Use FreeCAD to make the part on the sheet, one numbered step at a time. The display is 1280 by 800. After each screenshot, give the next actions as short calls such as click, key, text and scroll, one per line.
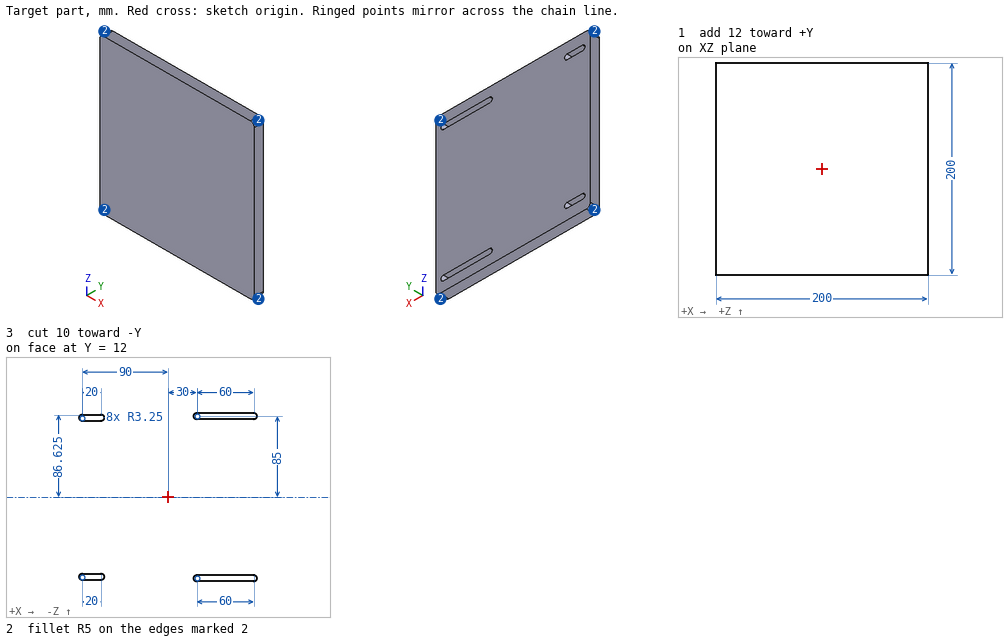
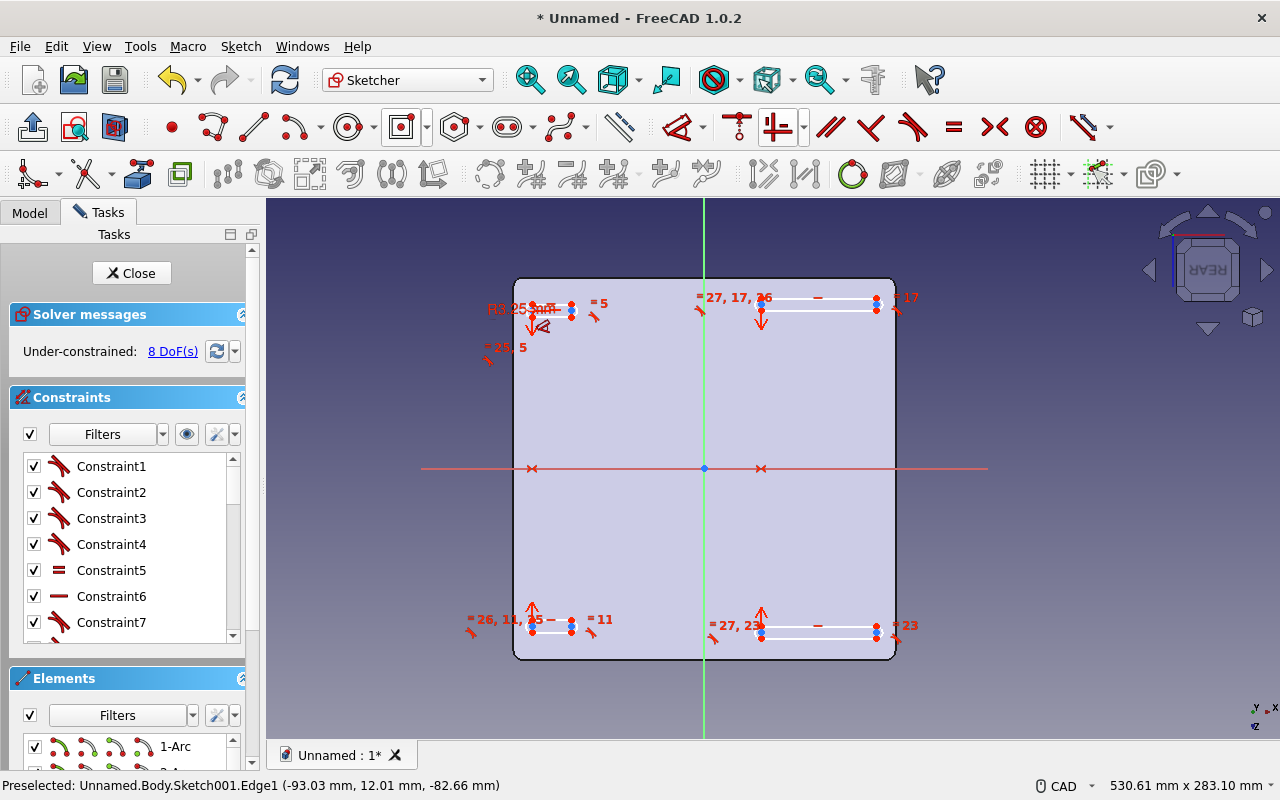
click(544, 305)
click(552, 271)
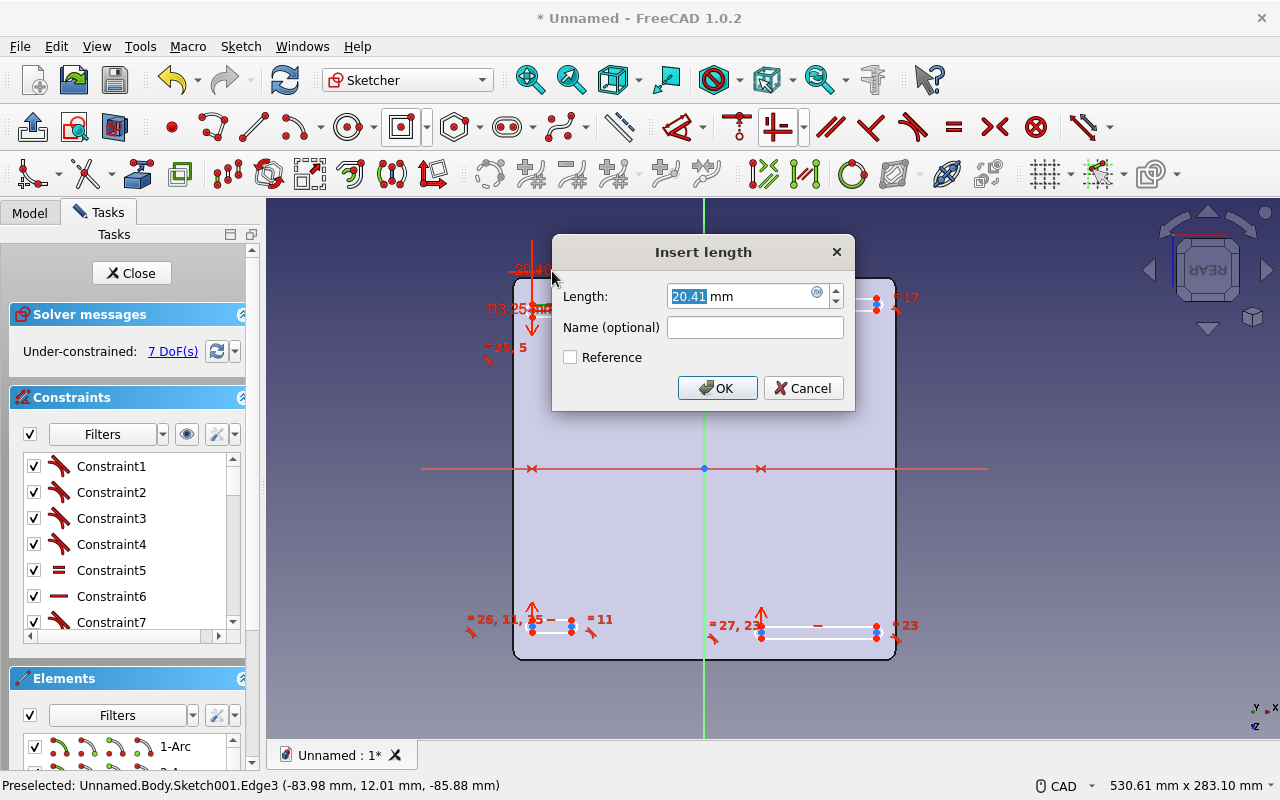
text(20)
key(Return)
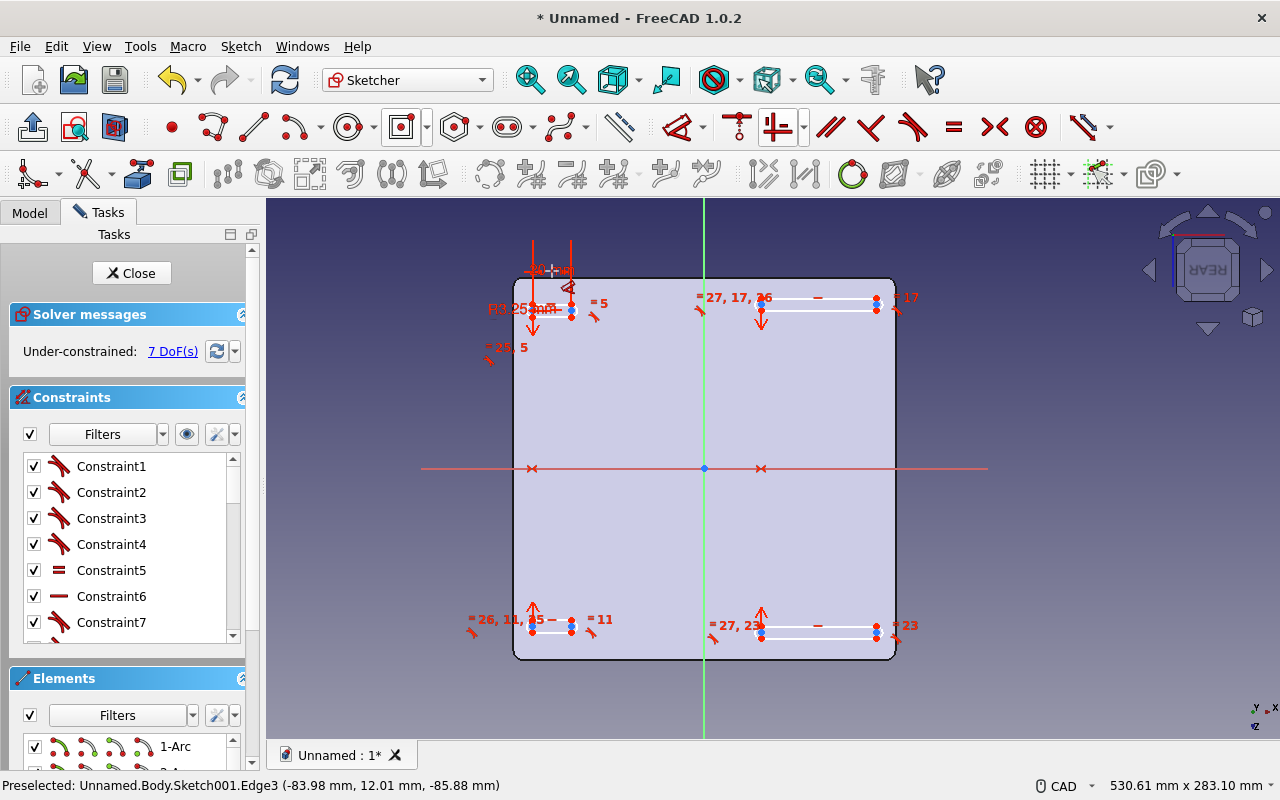
click(544, 620)
click(552, 654)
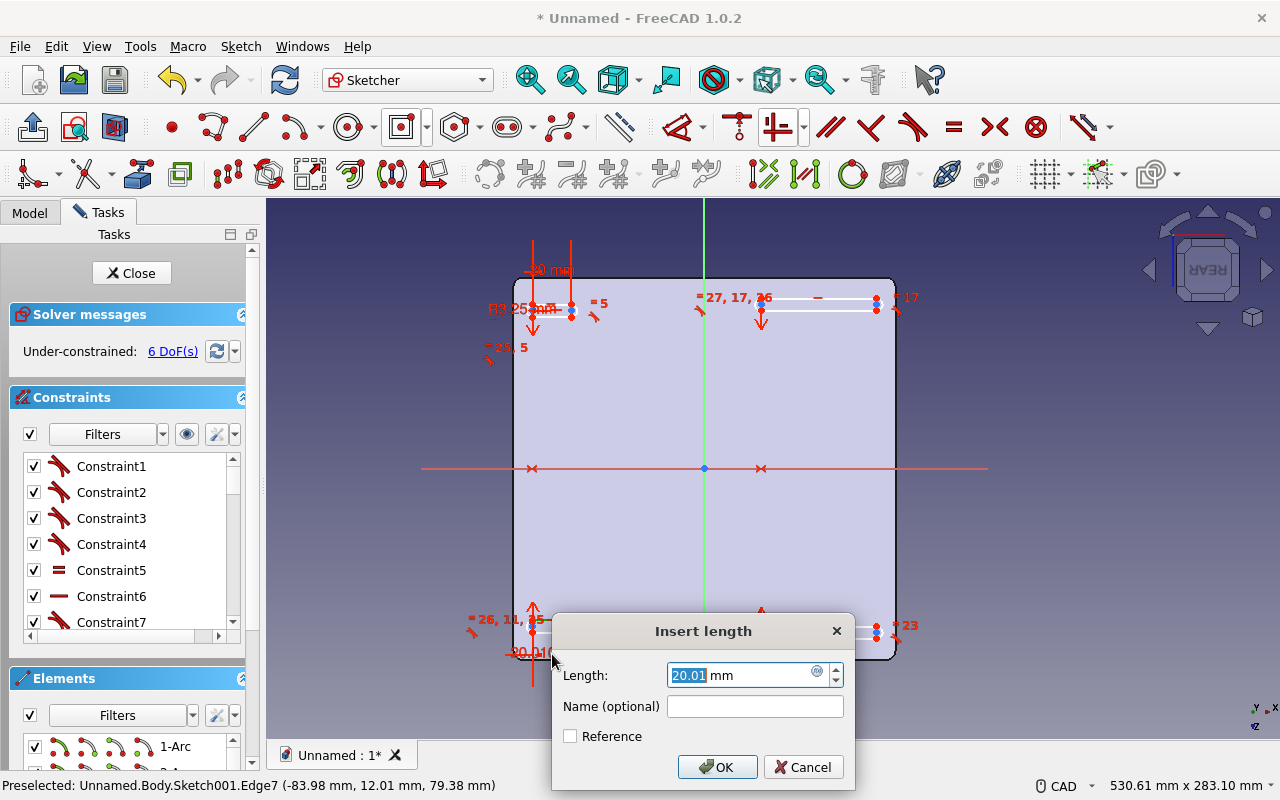
text(20)
key(Return)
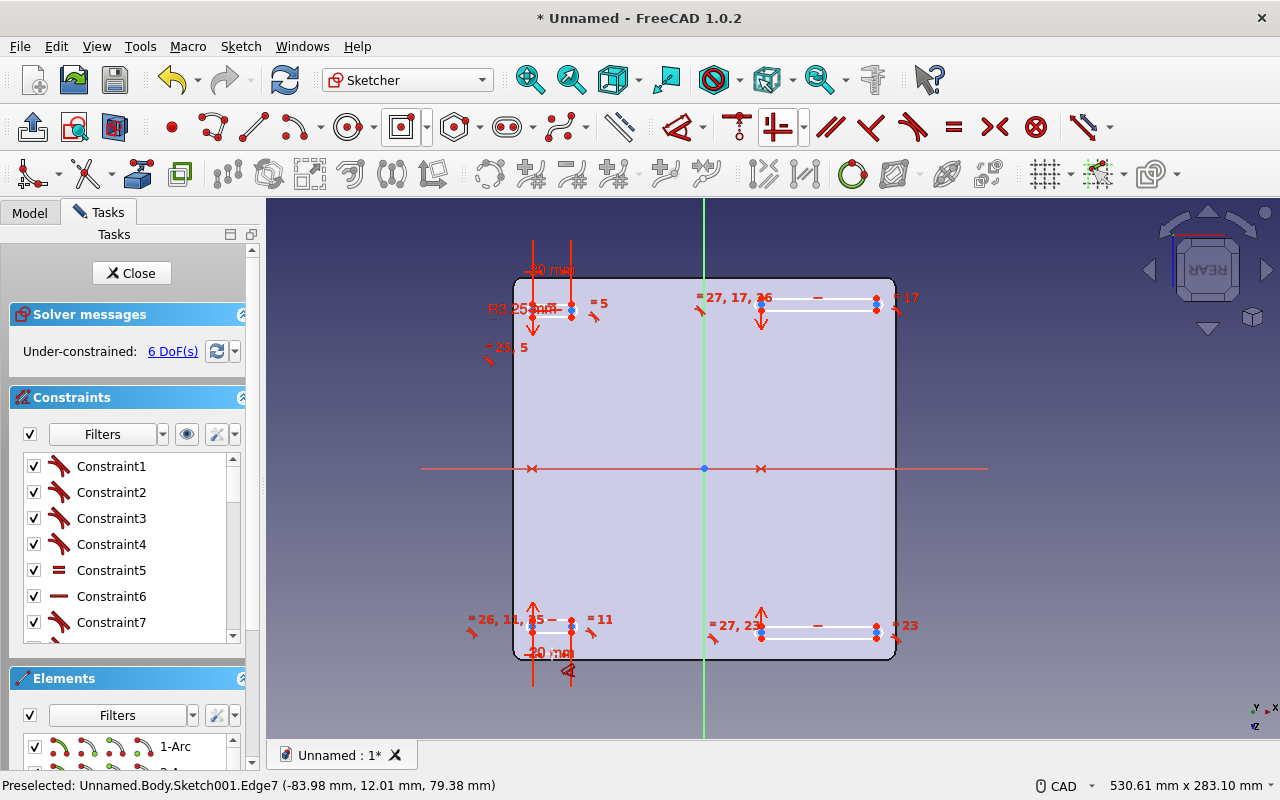
click(796, 299)
click(819, 265)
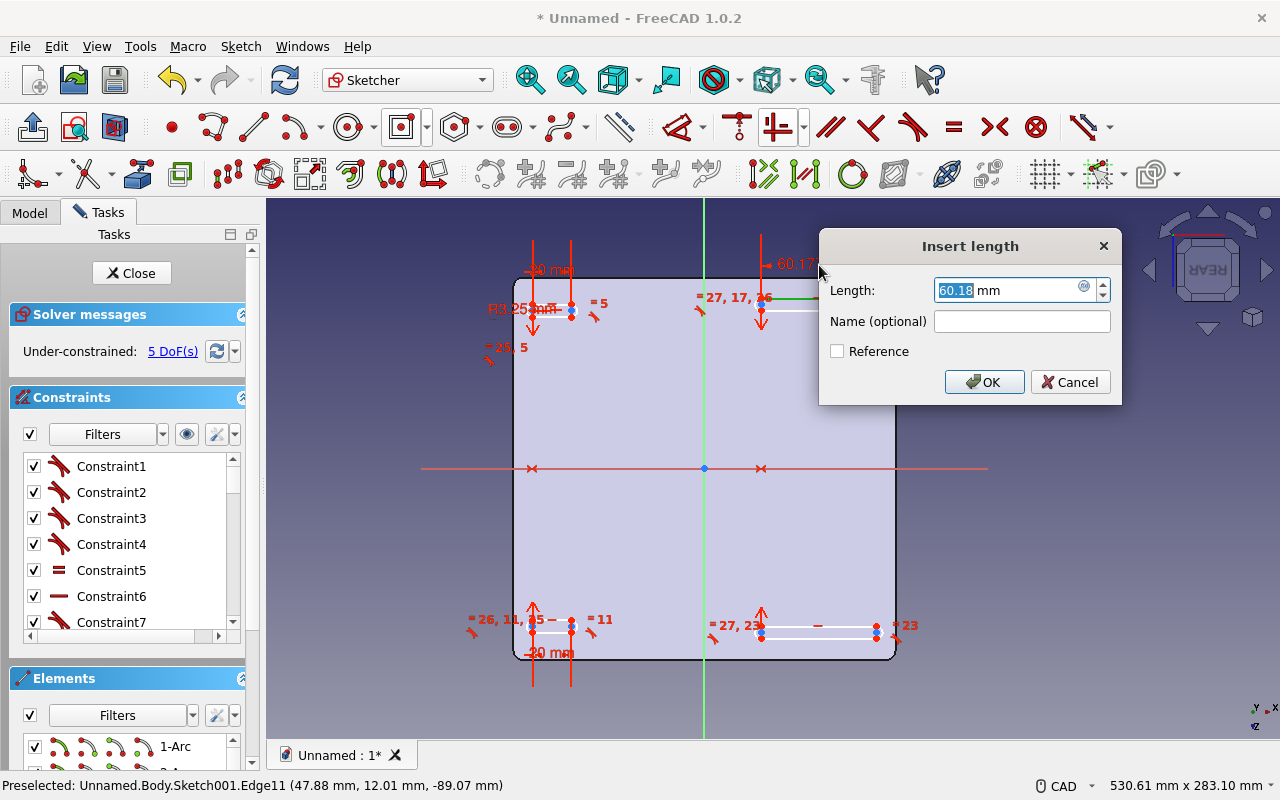
text(60)
key(Return)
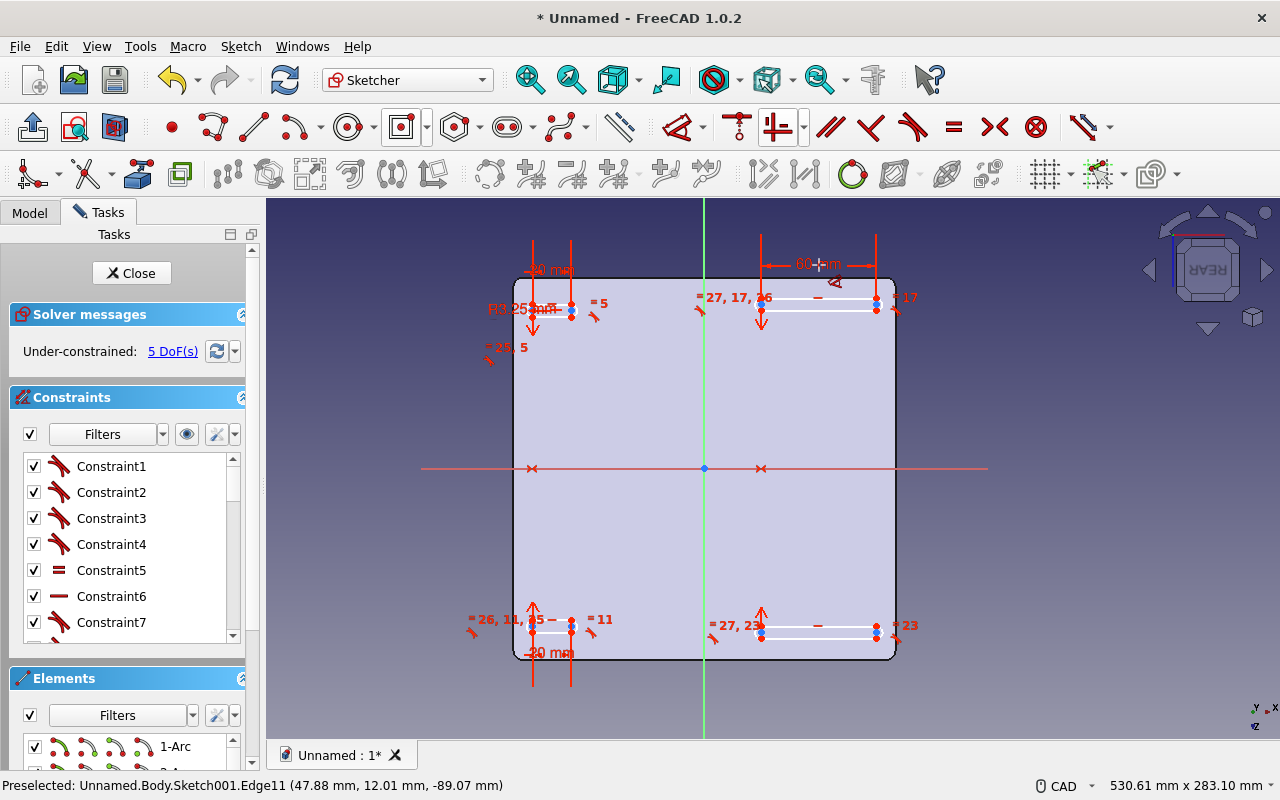
click(796, 627)
click(819, 661)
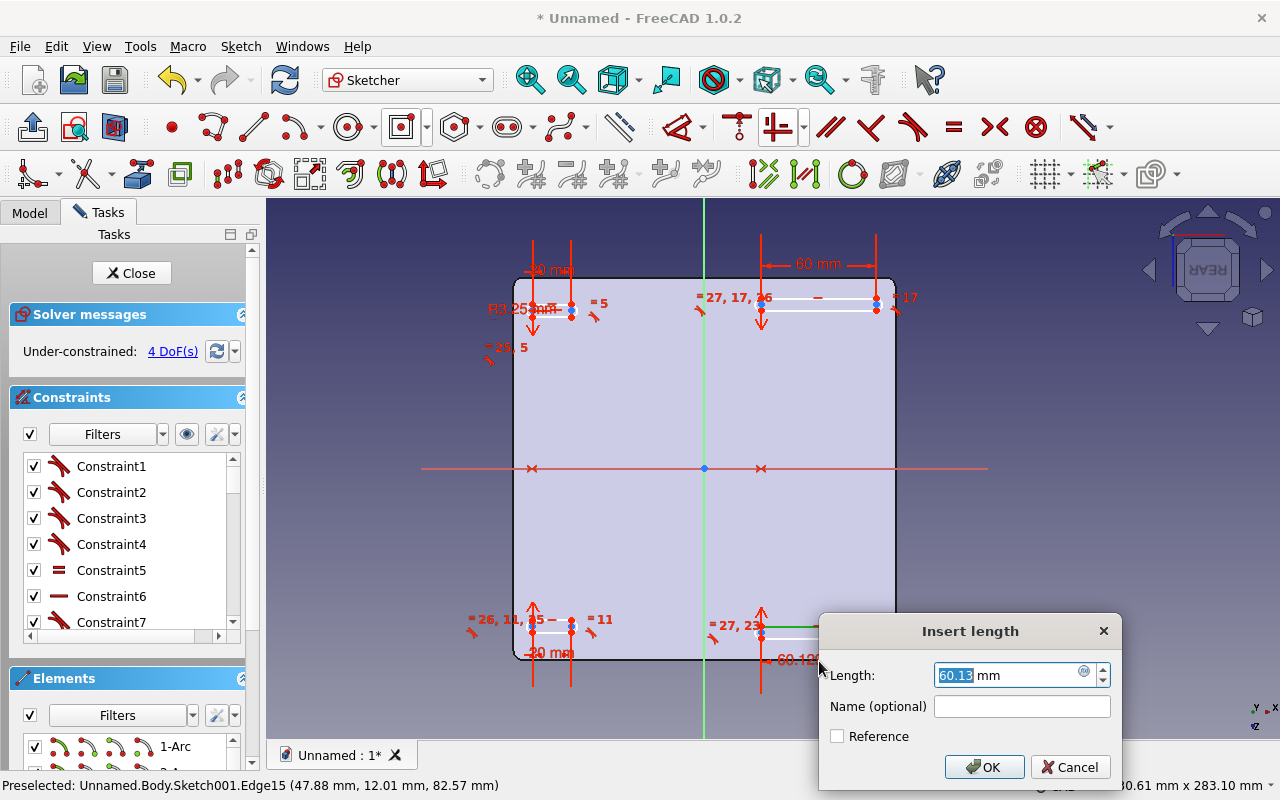
text(60)
key(Return)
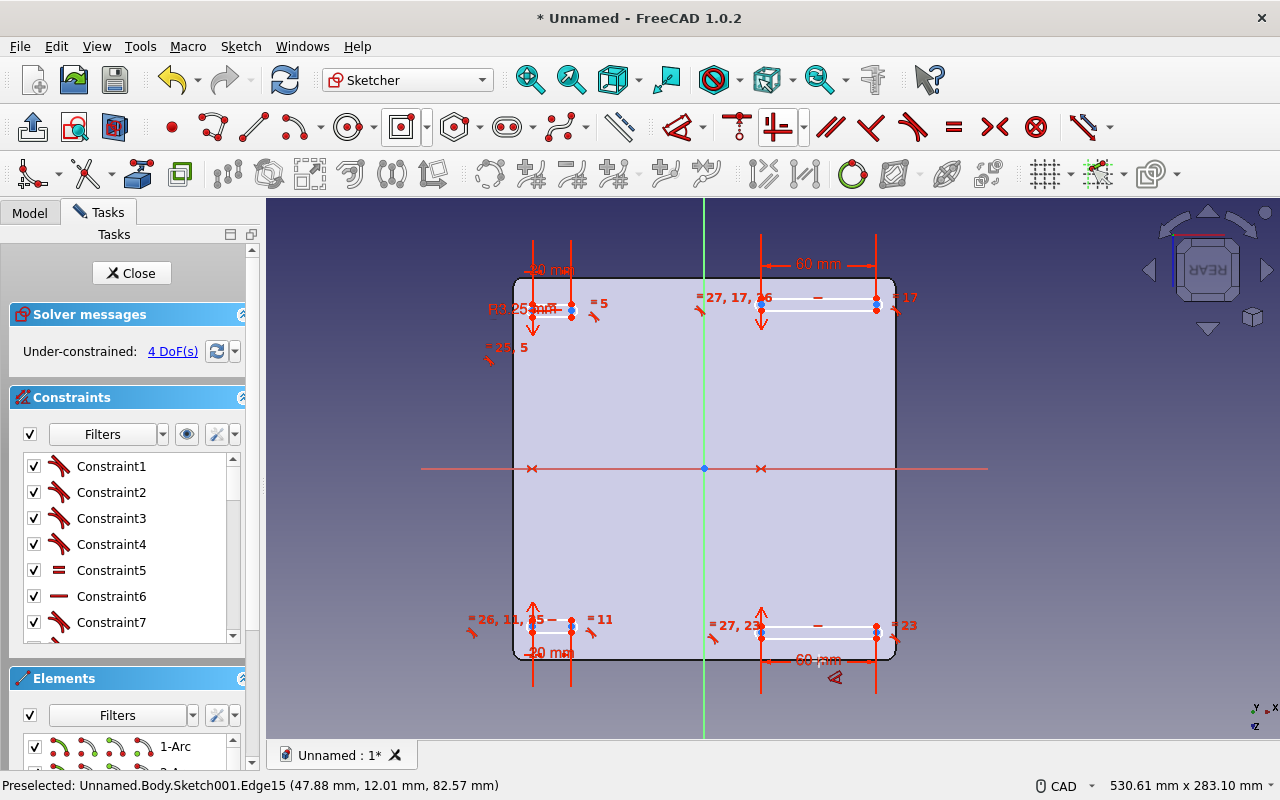
scroll(533, 305, up, 4)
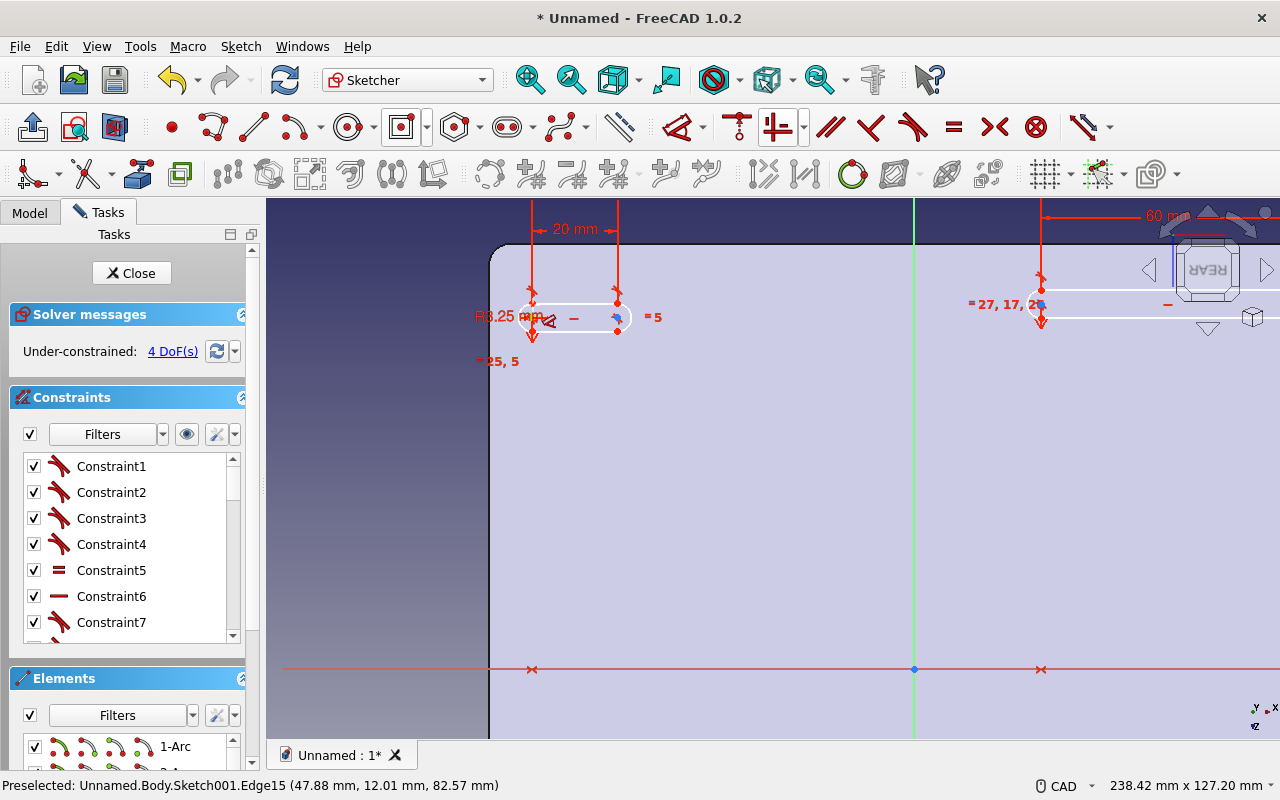
click(532, 304)
click(723, 270)